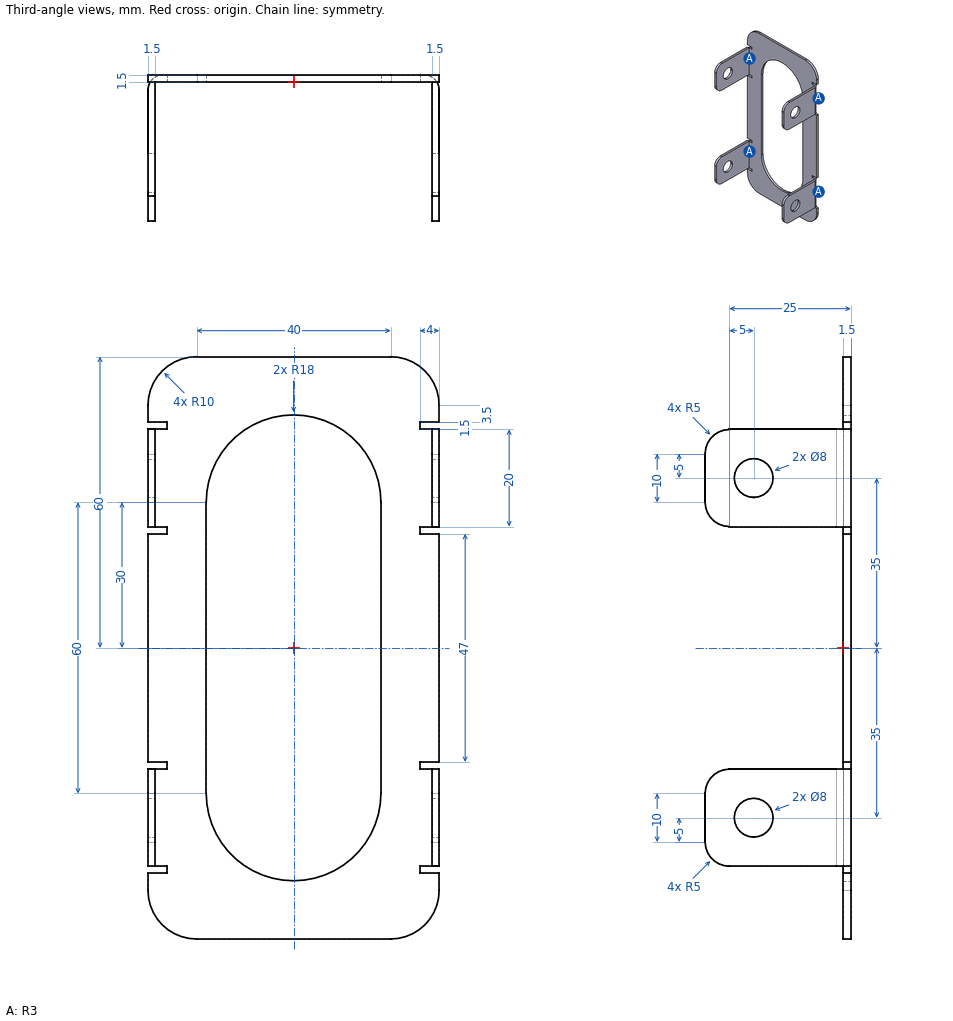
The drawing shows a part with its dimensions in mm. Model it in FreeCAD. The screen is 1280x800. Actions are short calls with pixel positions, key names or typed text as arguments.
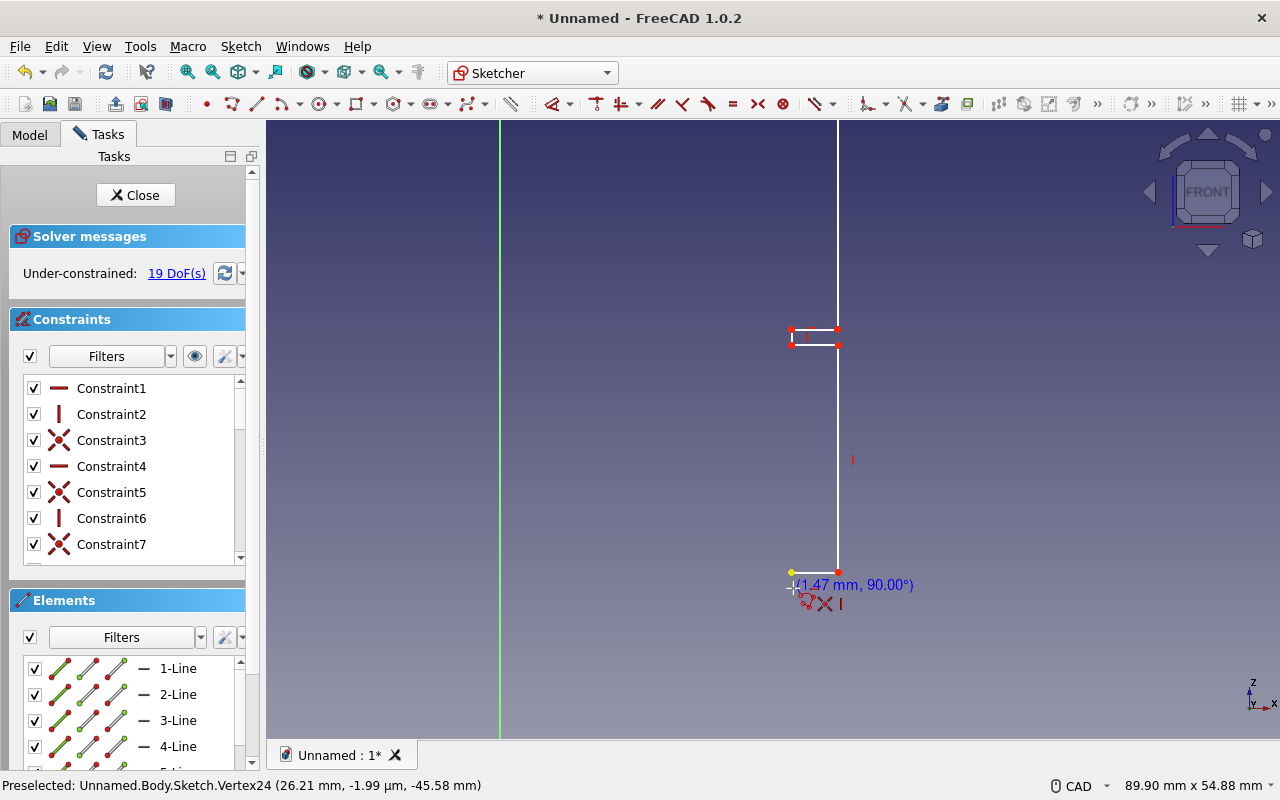
click(792, 587)
click(838, 587)
click(838, 626)
right_click(838, 626)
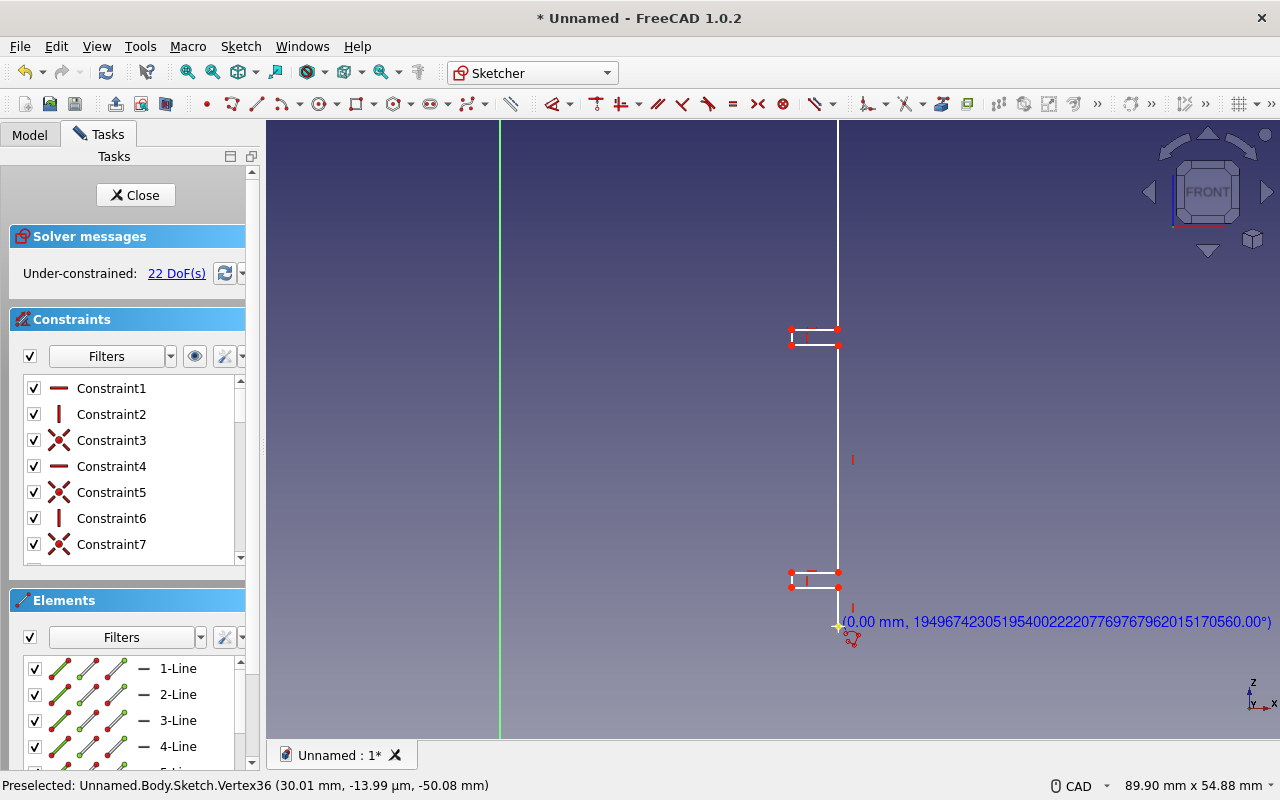
click(257, 104)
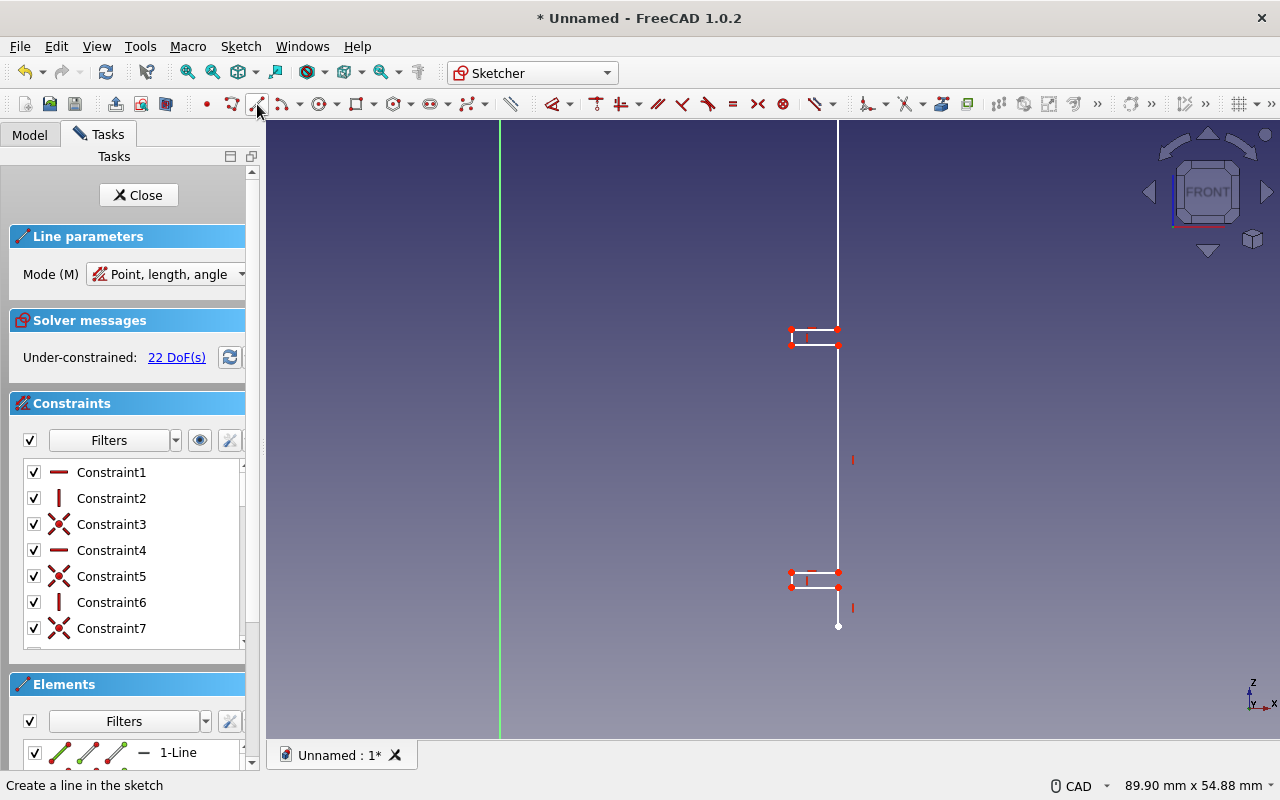
scroll(793, 588, down, 6)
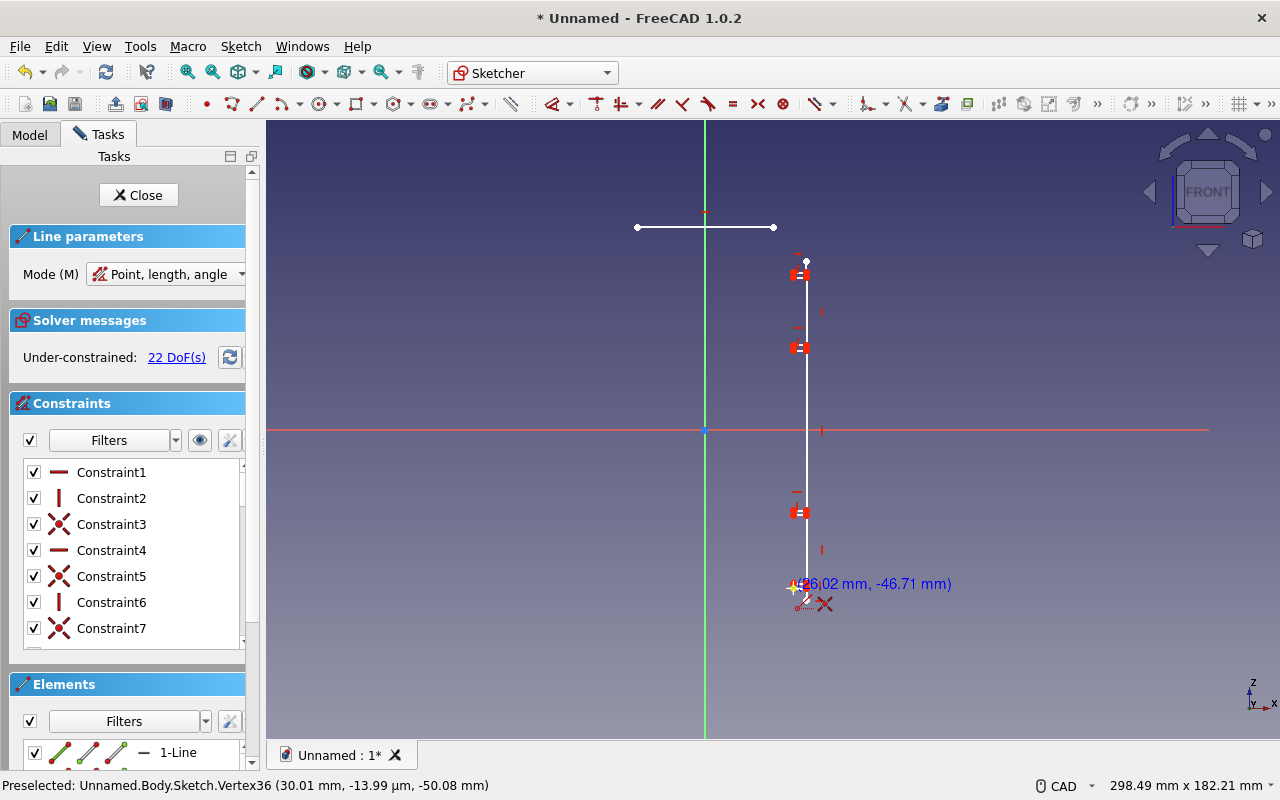
click(773, 634)
click(637, 634)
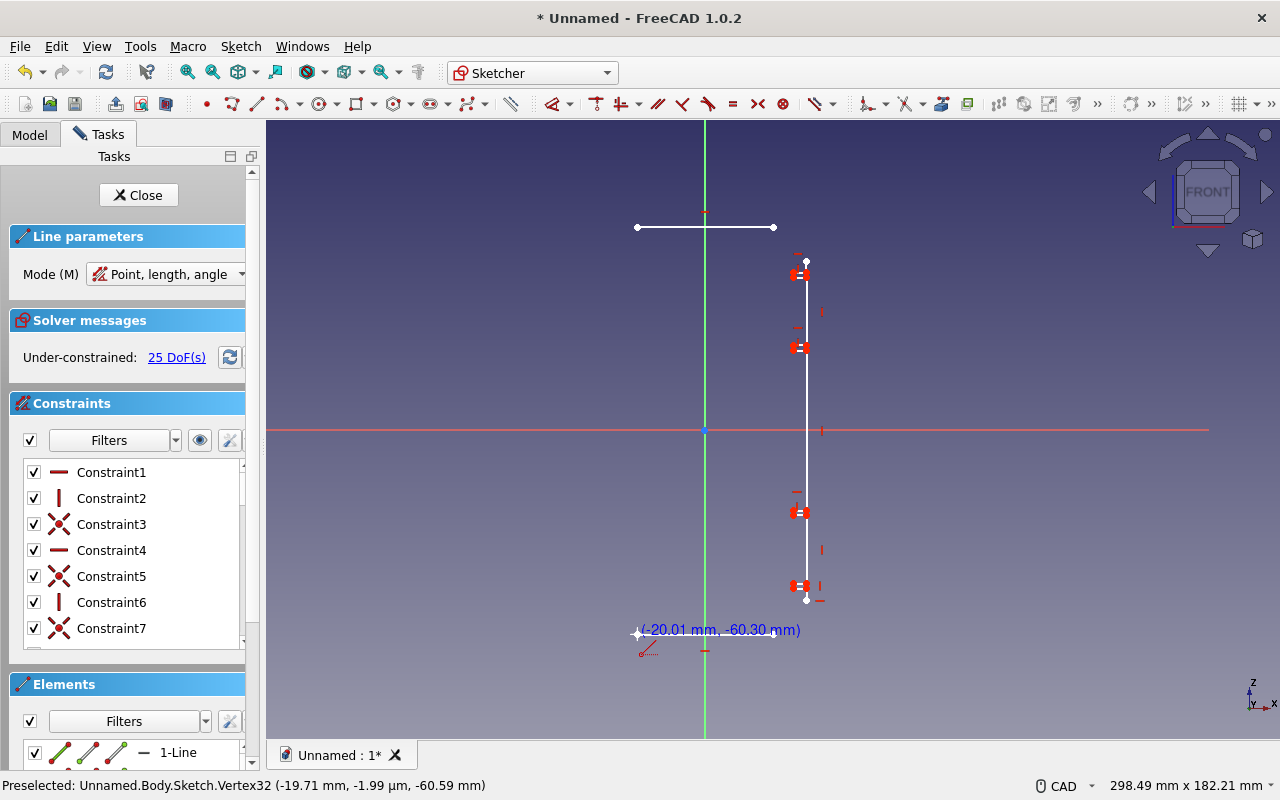
key(g)
key(m)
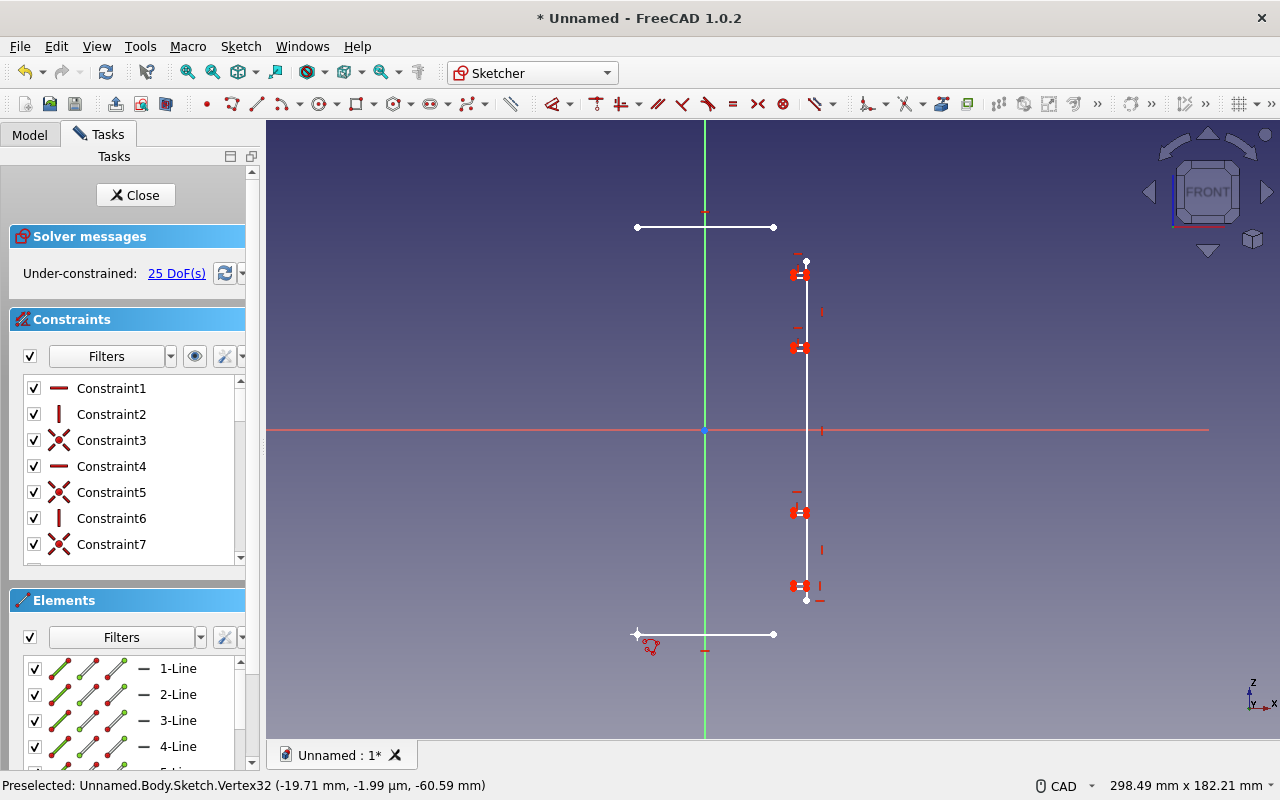
click(603, 600)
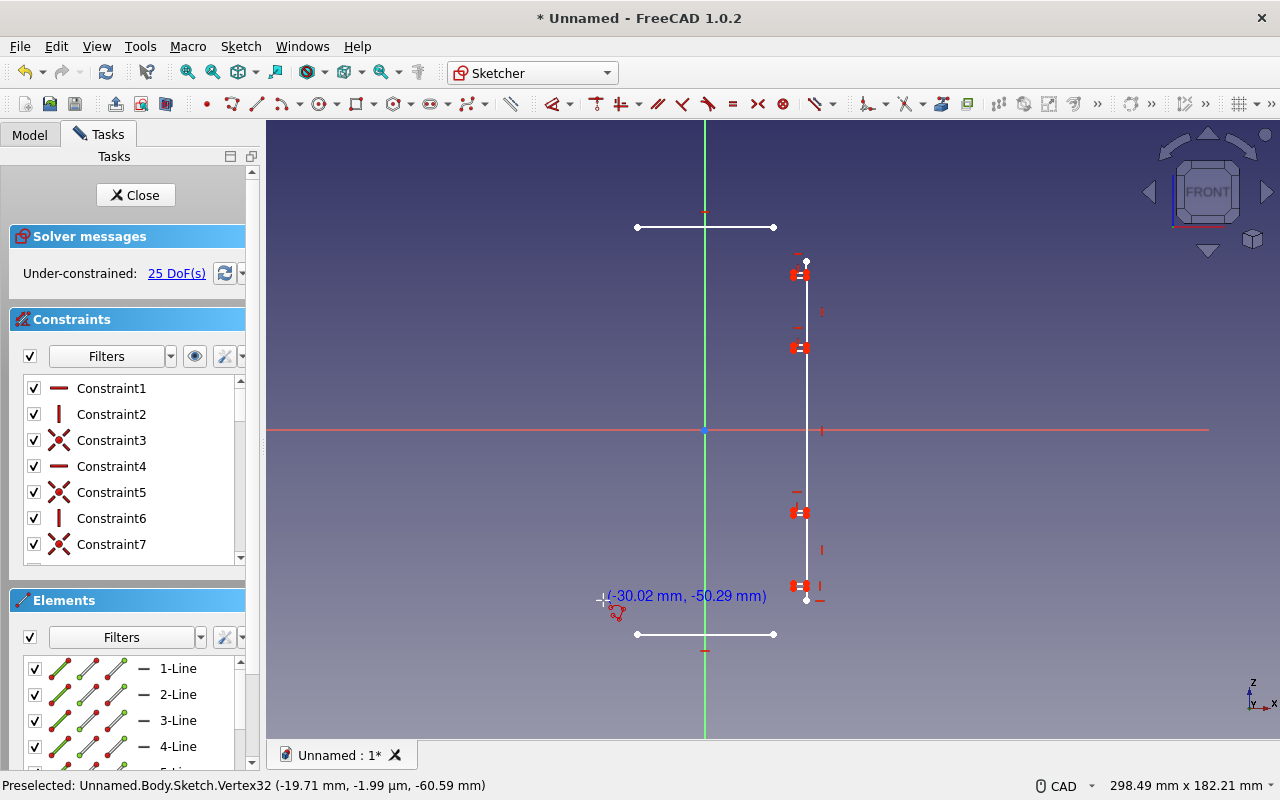
scroll(603, 588, up, 2)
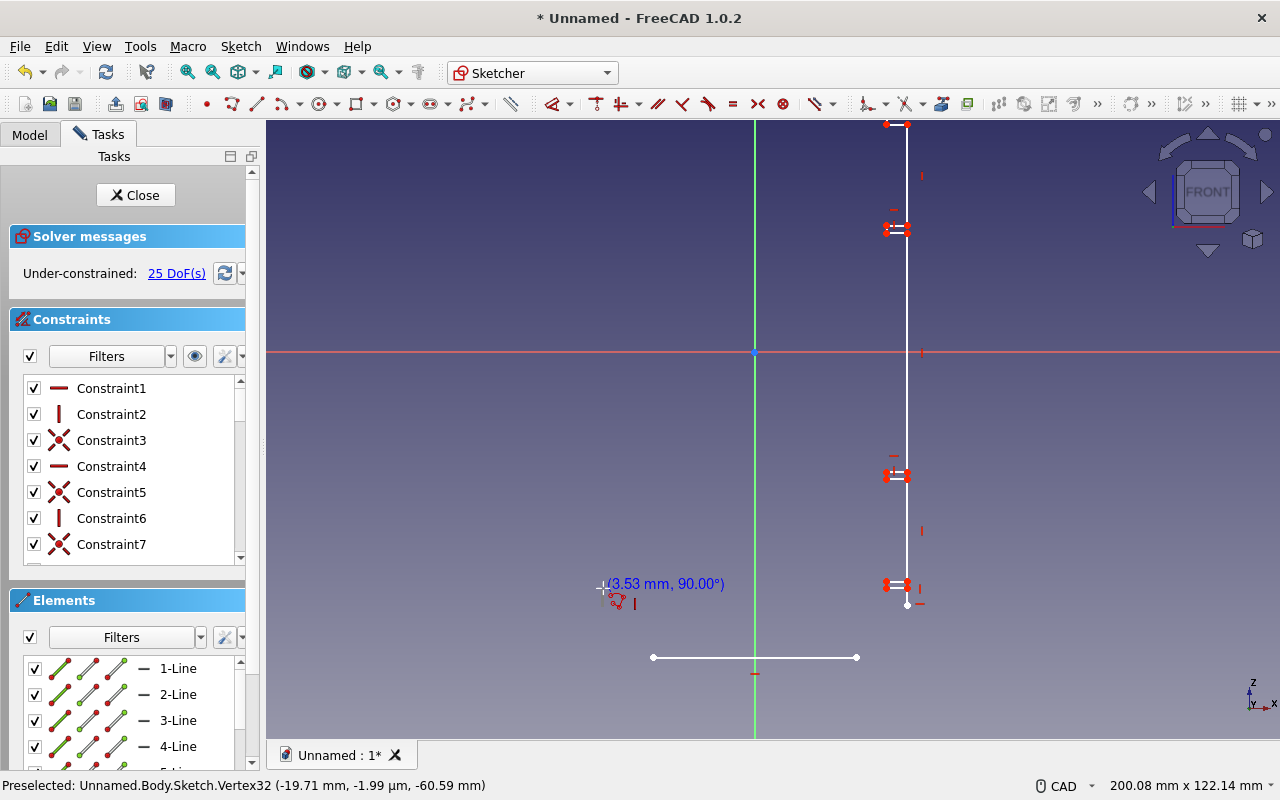
click(603, 588)
click(623, 588)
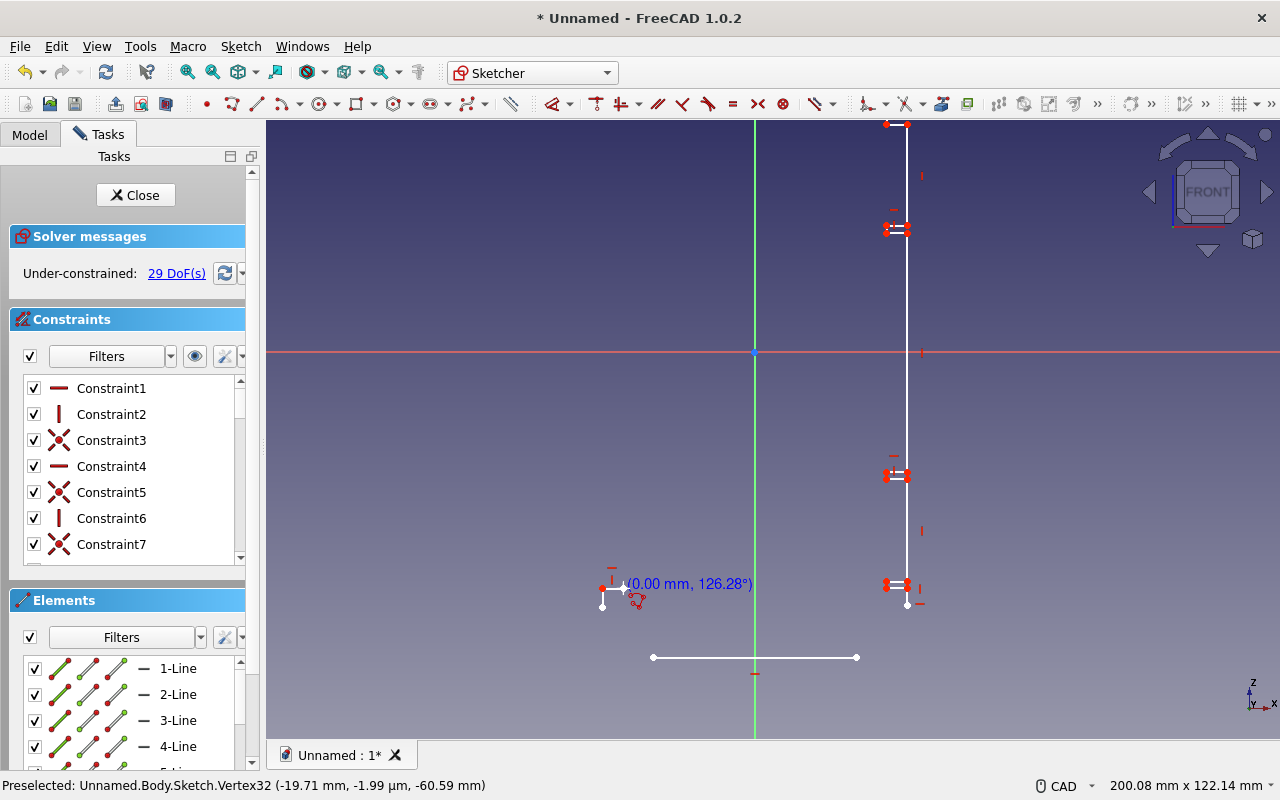
scroll(623, 580, up, 4)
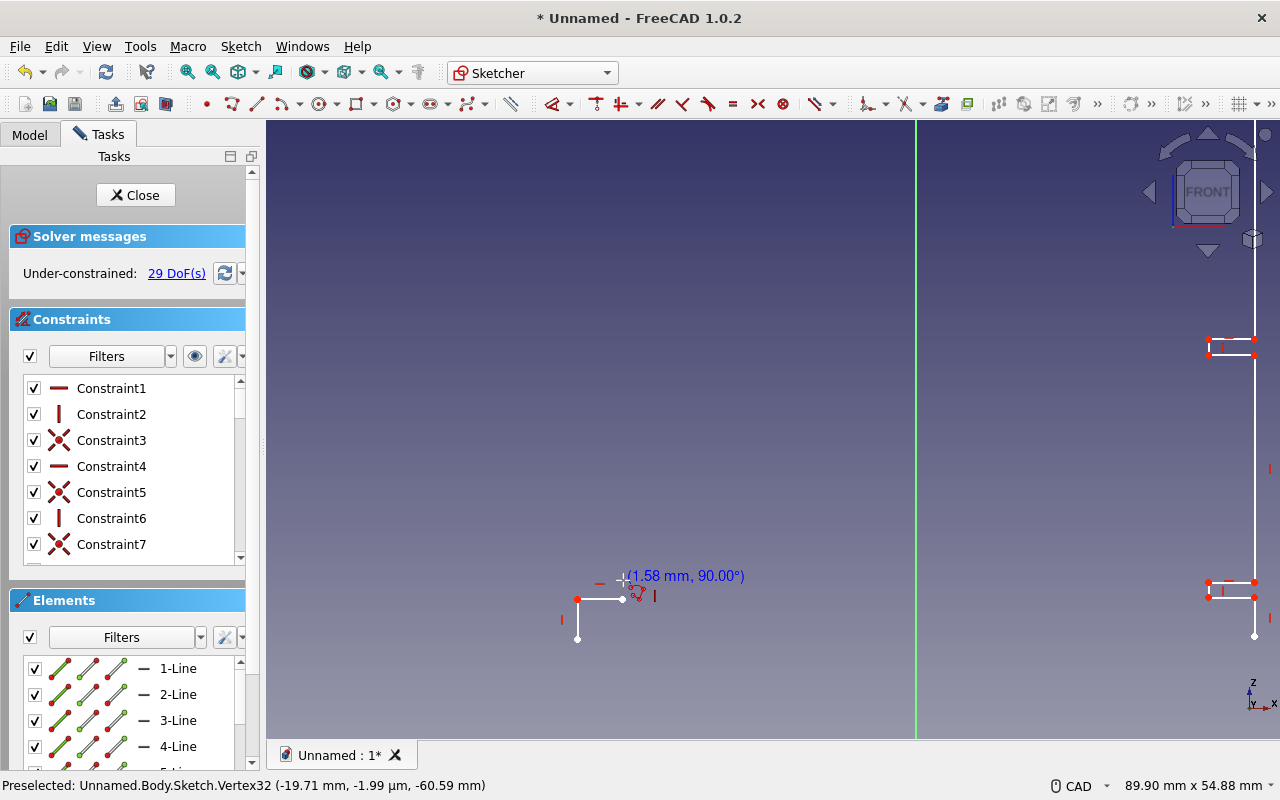
click(623, 580)
click(578, 580)
click(578, 354)
click(623, 354)
click(623, 337)
click(578, 337)